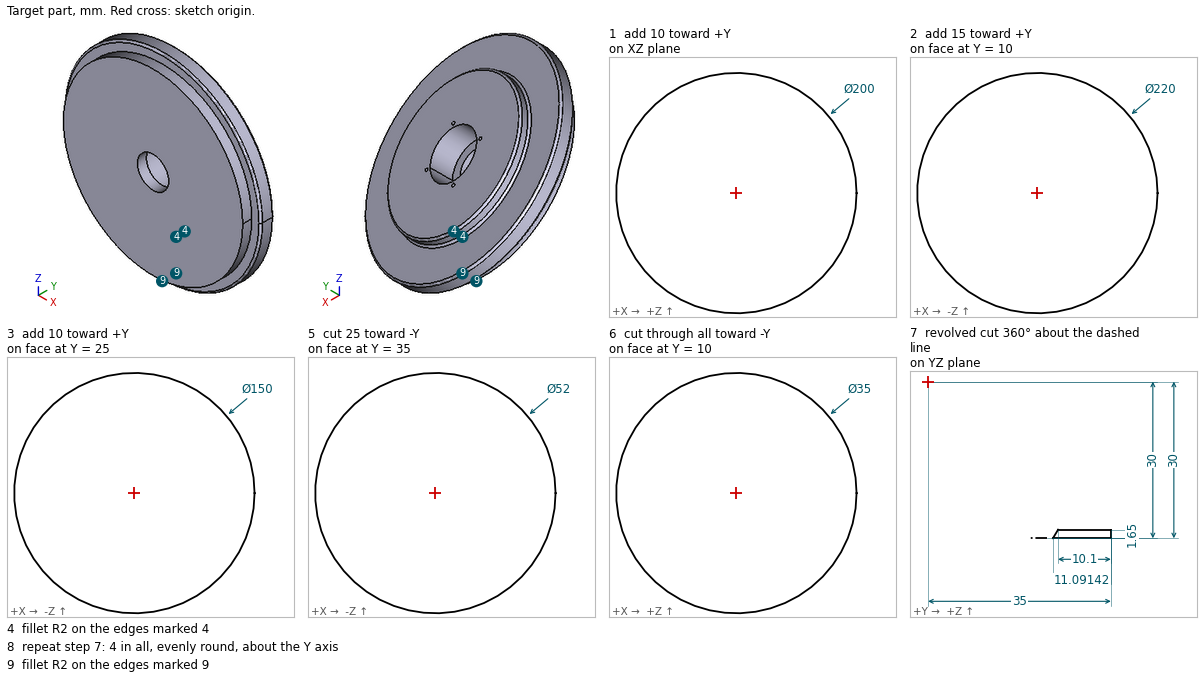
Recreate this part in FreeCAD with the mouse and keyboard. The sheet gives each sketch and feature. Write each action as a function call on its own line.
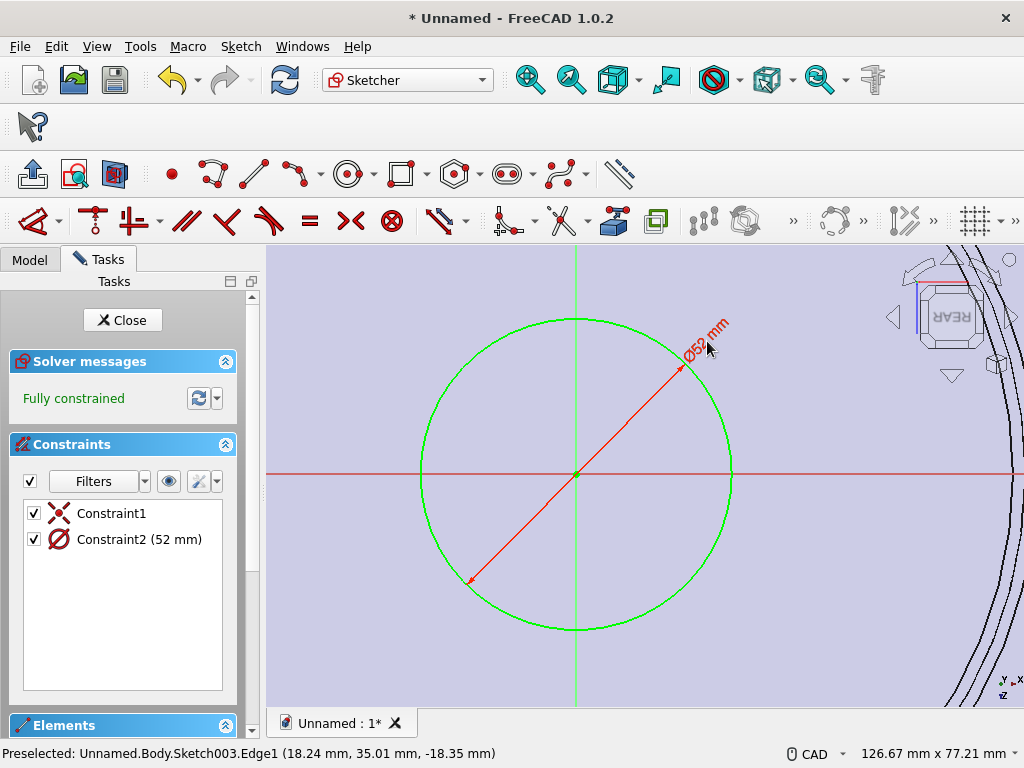
click(123, 320)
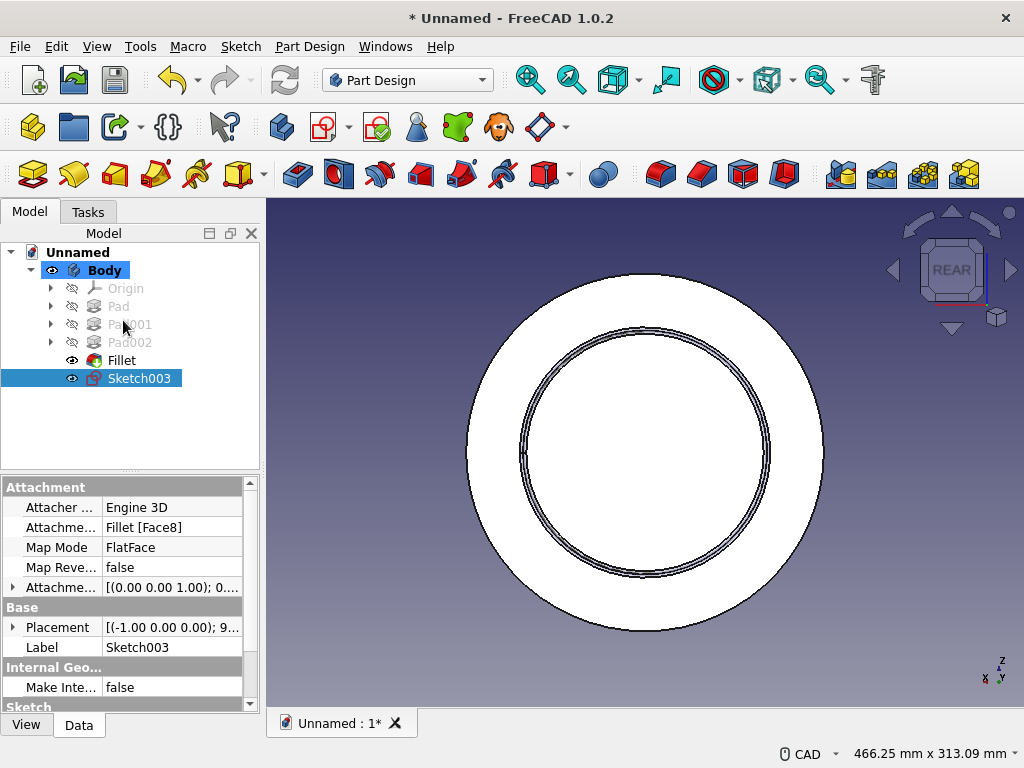
click(298, 174)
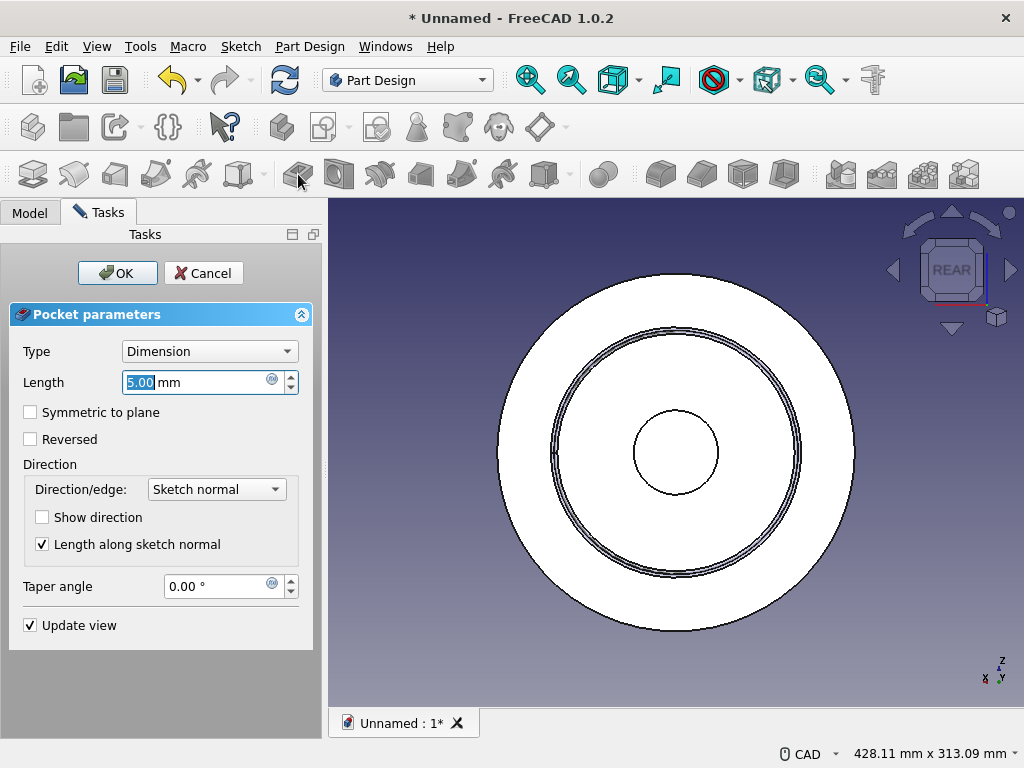
text(25)
key(Tab)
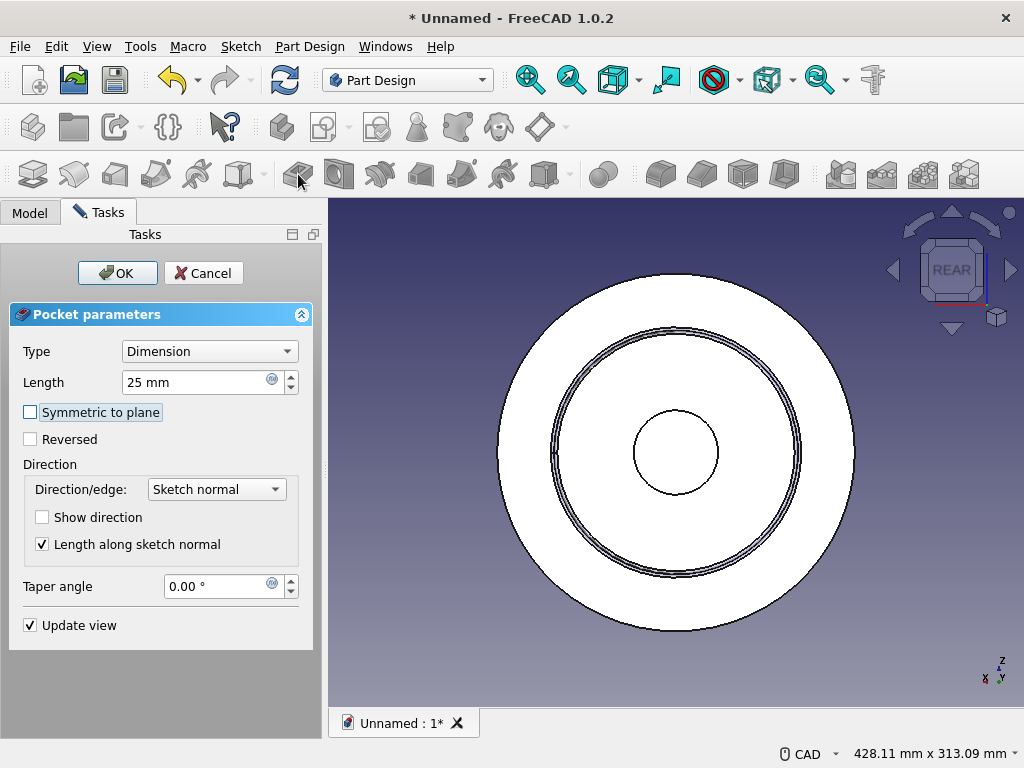
click(118, 273)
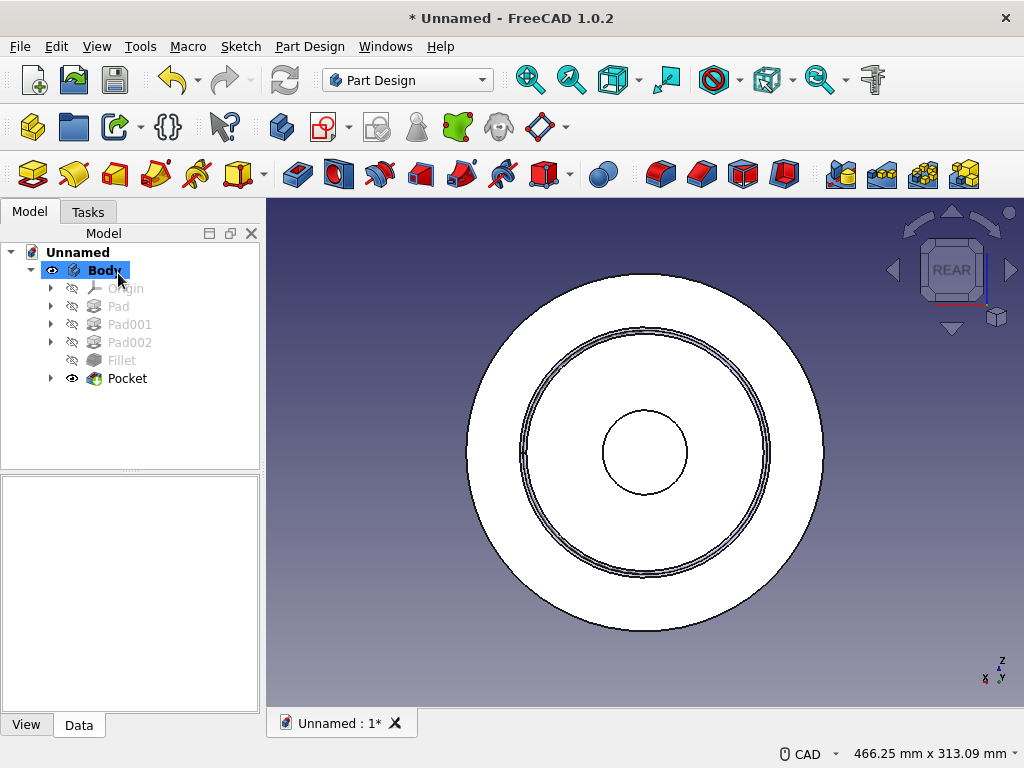
key(0)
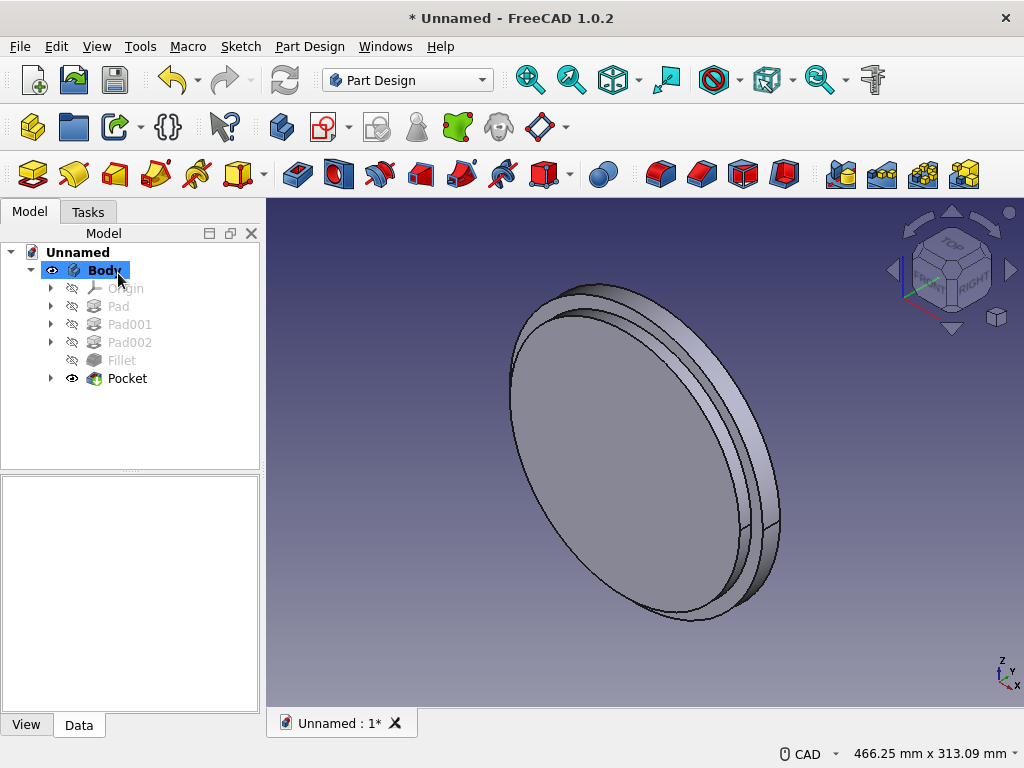
click(710, 612)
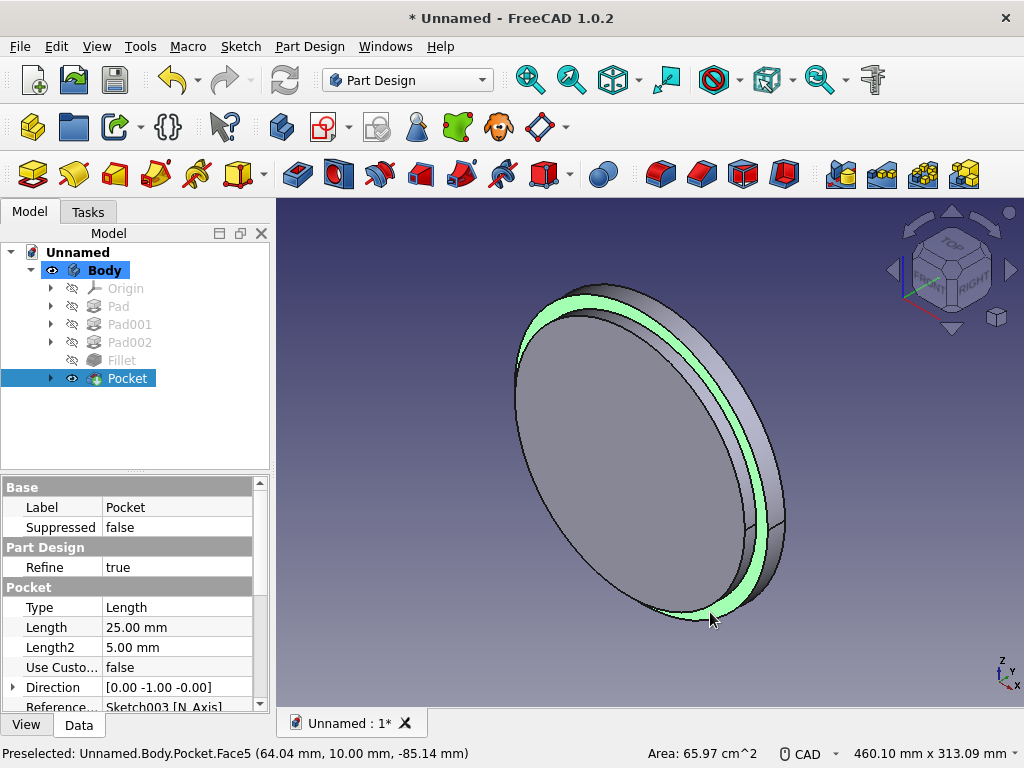
click(322, 128)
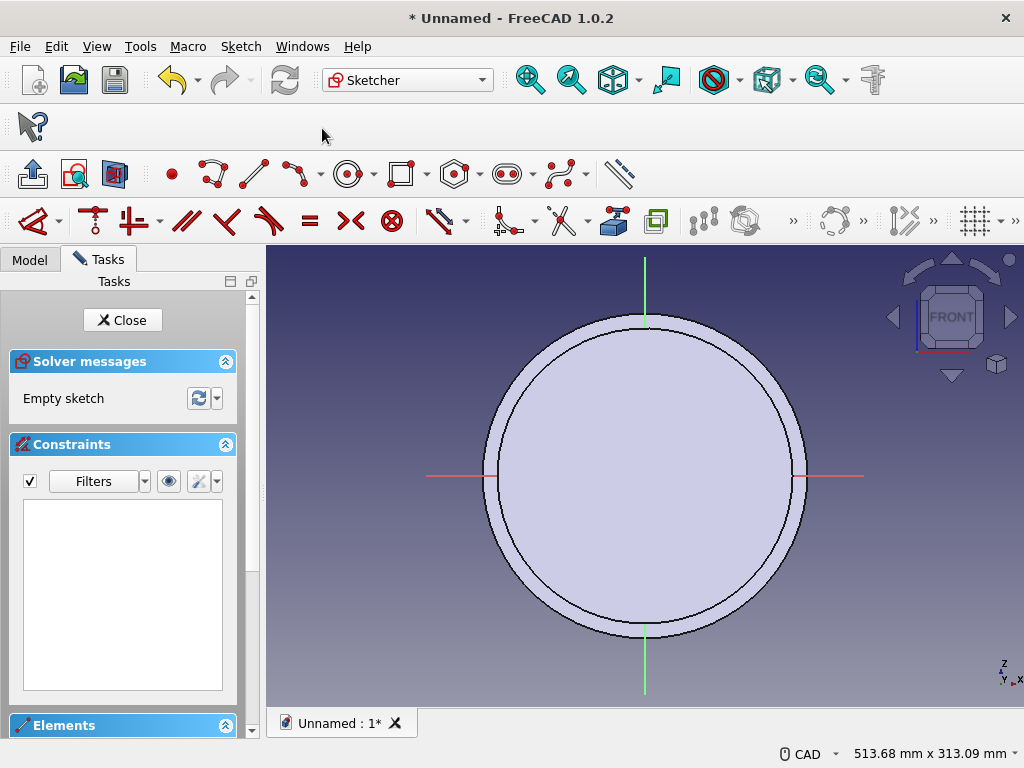
click(115, 174)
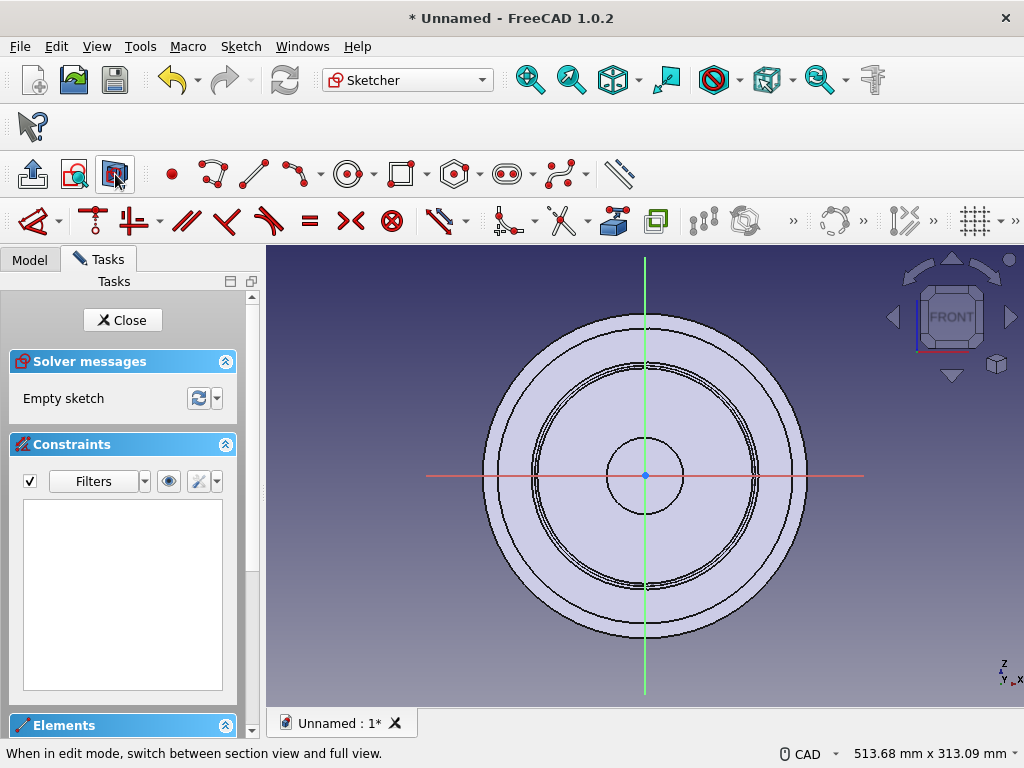
scroll(659, 476, up, 9)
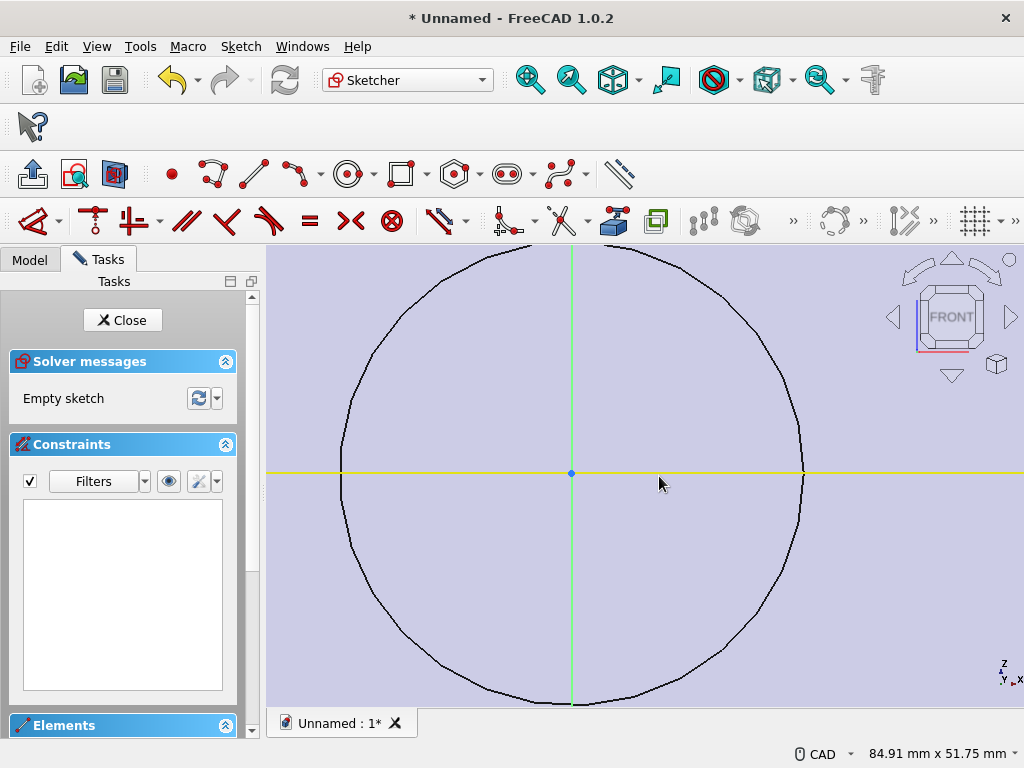
click(348, 174)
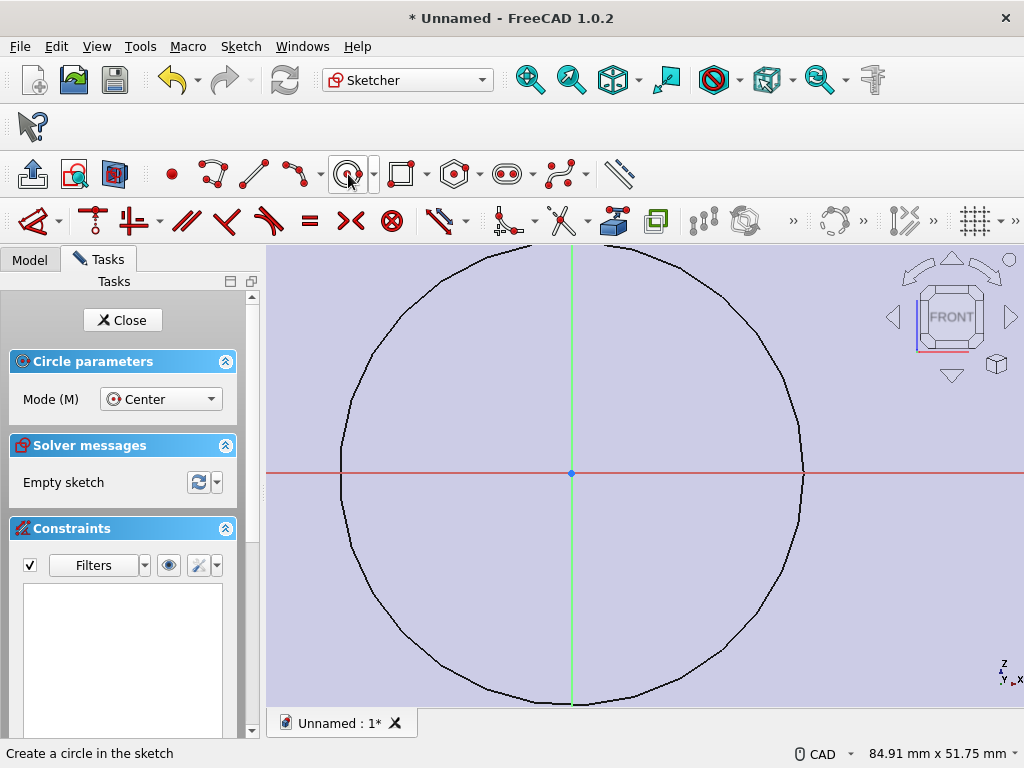
click(572, 473)
click(682, 363)
key(Escape)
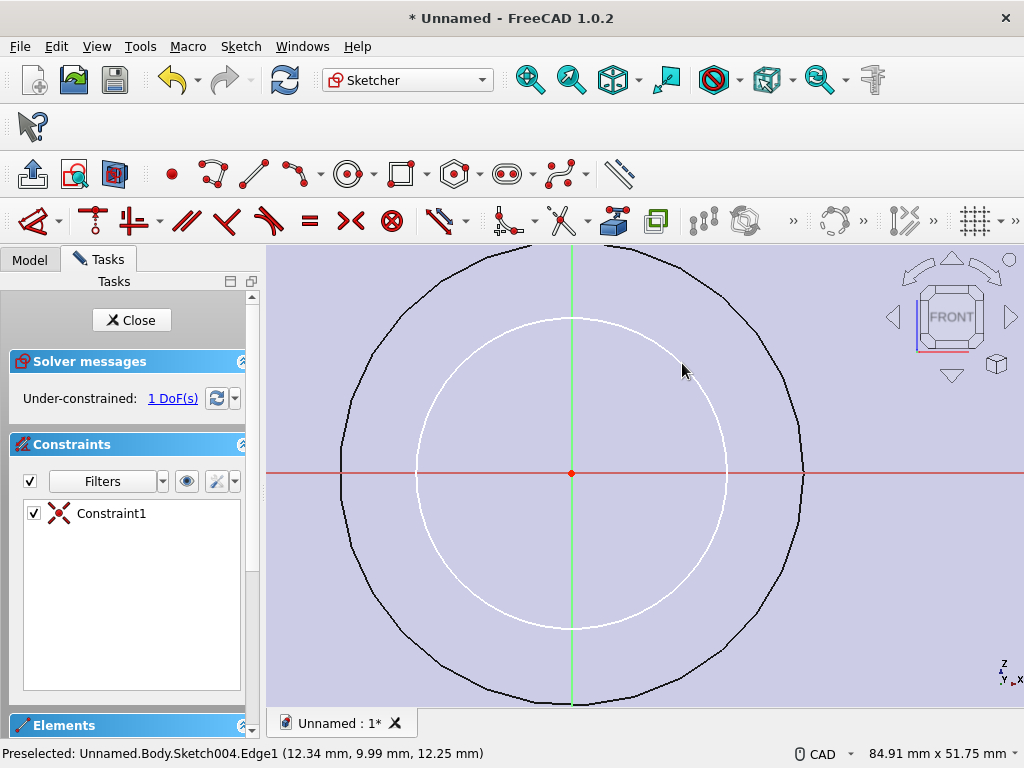
click(32, 222)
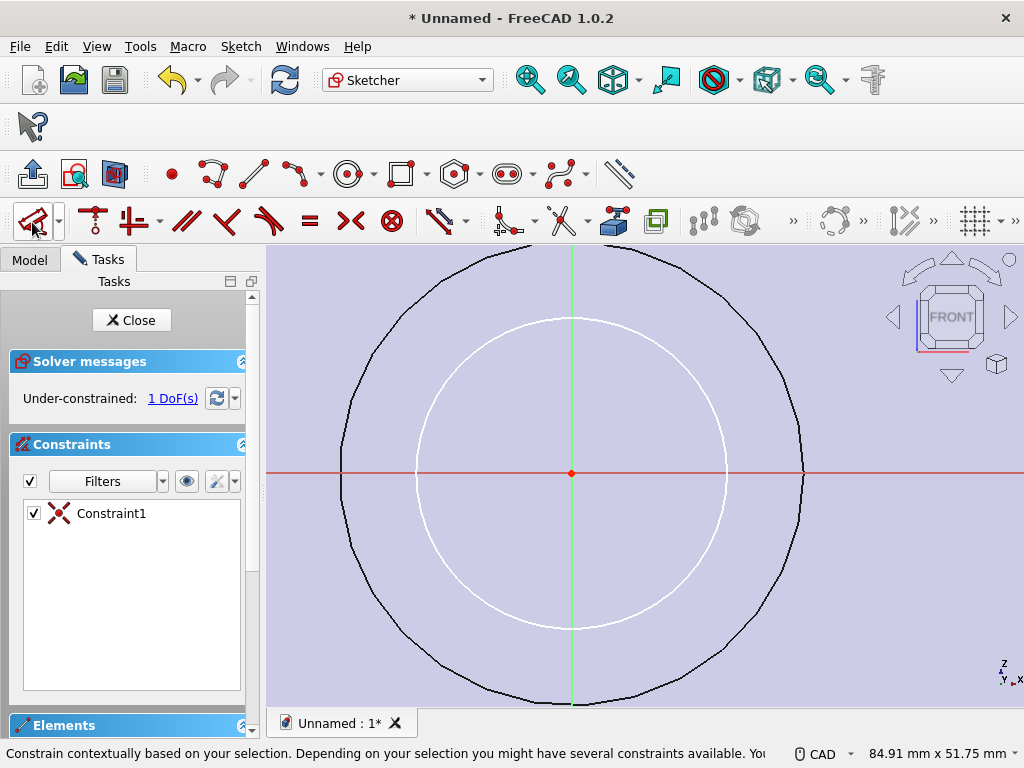
click(681, 363)
click(704, 340)